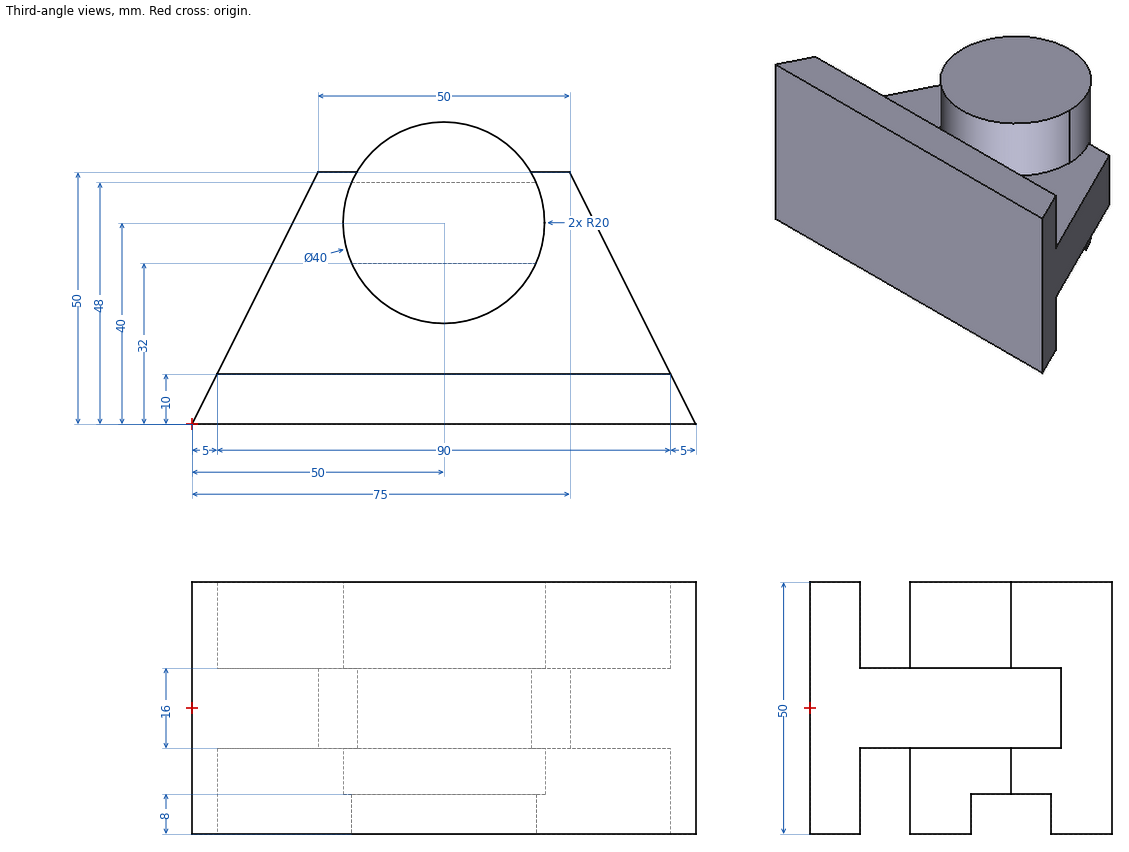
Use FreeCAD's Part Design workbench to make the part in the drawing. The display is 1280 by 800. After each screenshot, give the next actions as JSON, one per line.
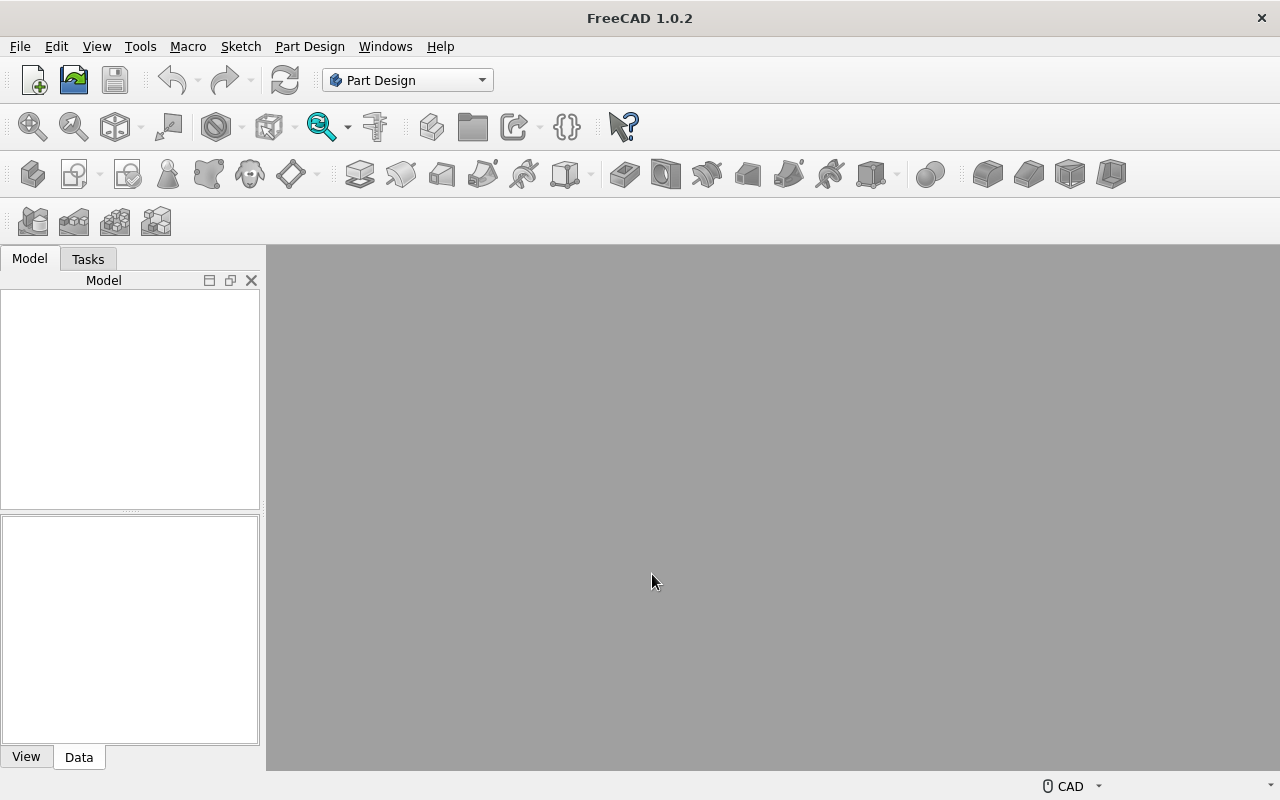
{"action": "left_click", "coordinate": [33, 80]}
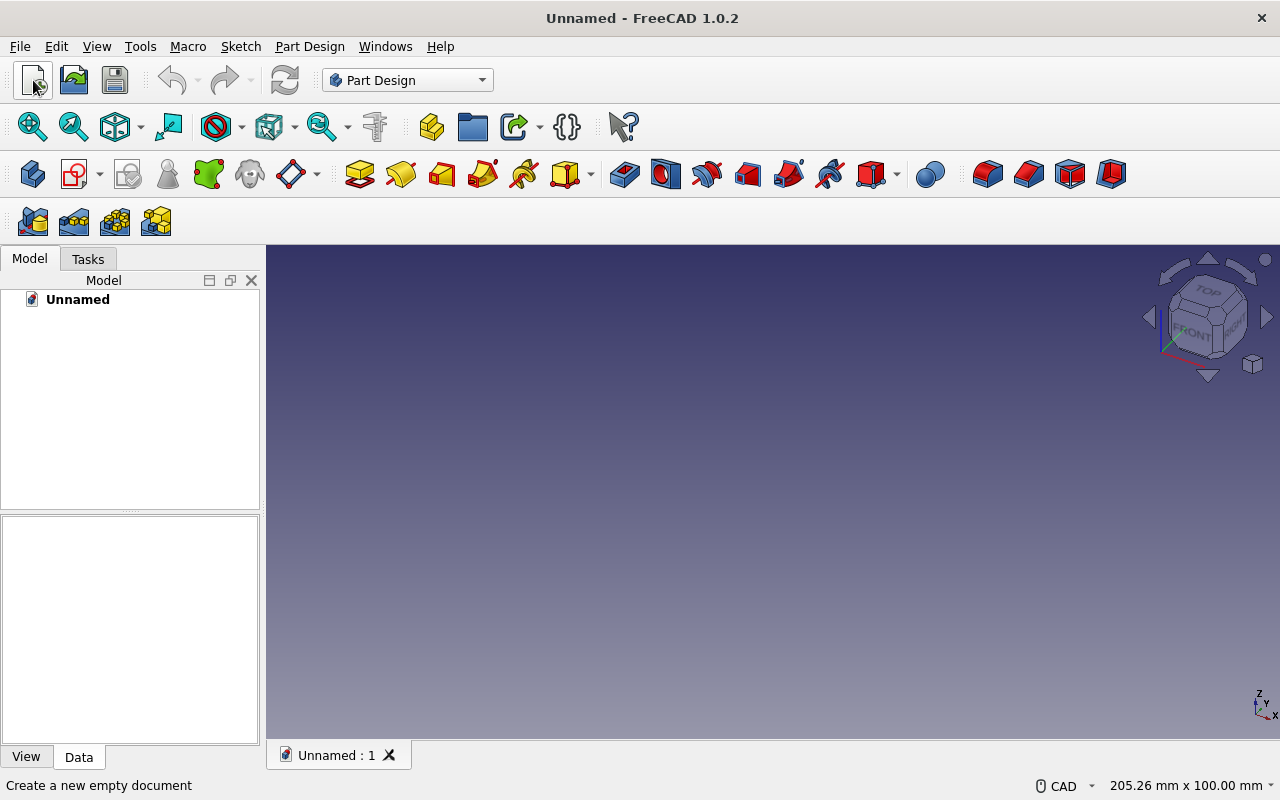
{"action": "left_click", "coordinate": [74, 174]}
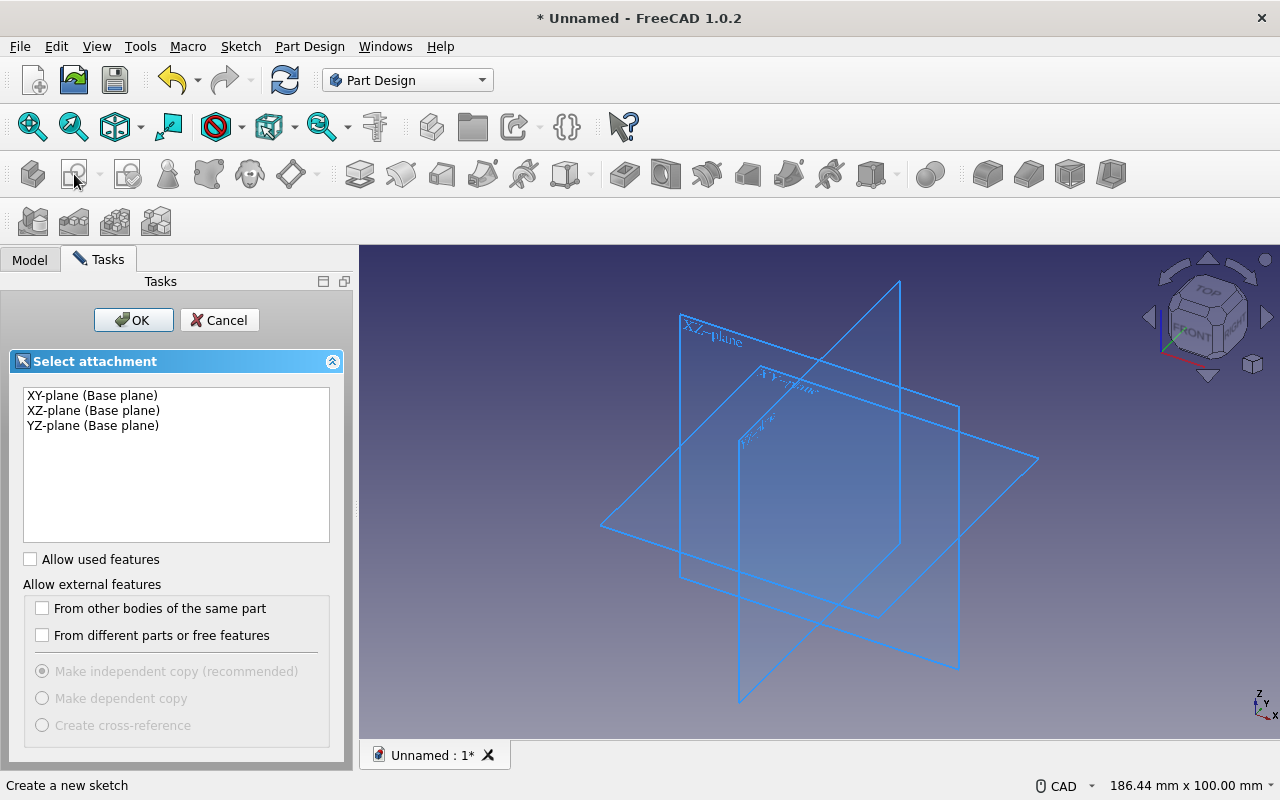
{"action": "left_click", "coordinate": [84, 396]}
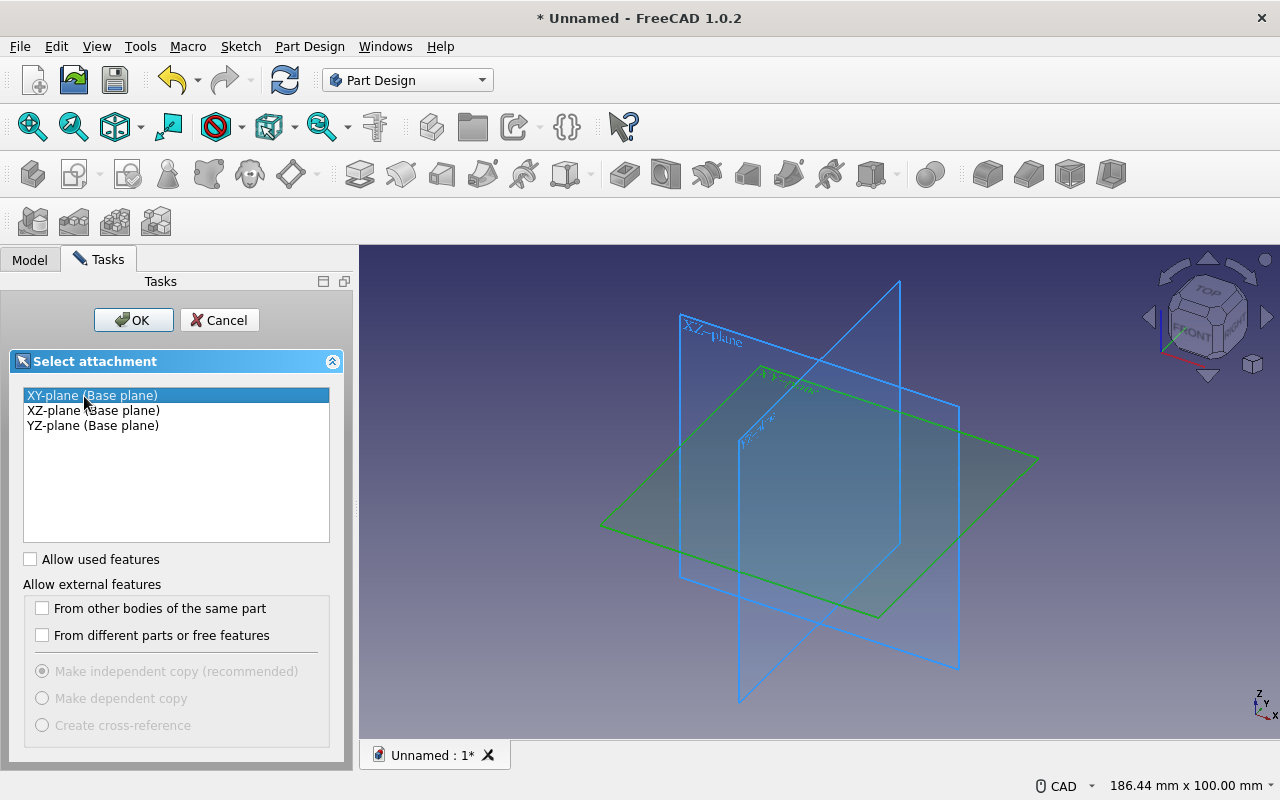
{"action": "left_click", "coordinate": [134, 320]}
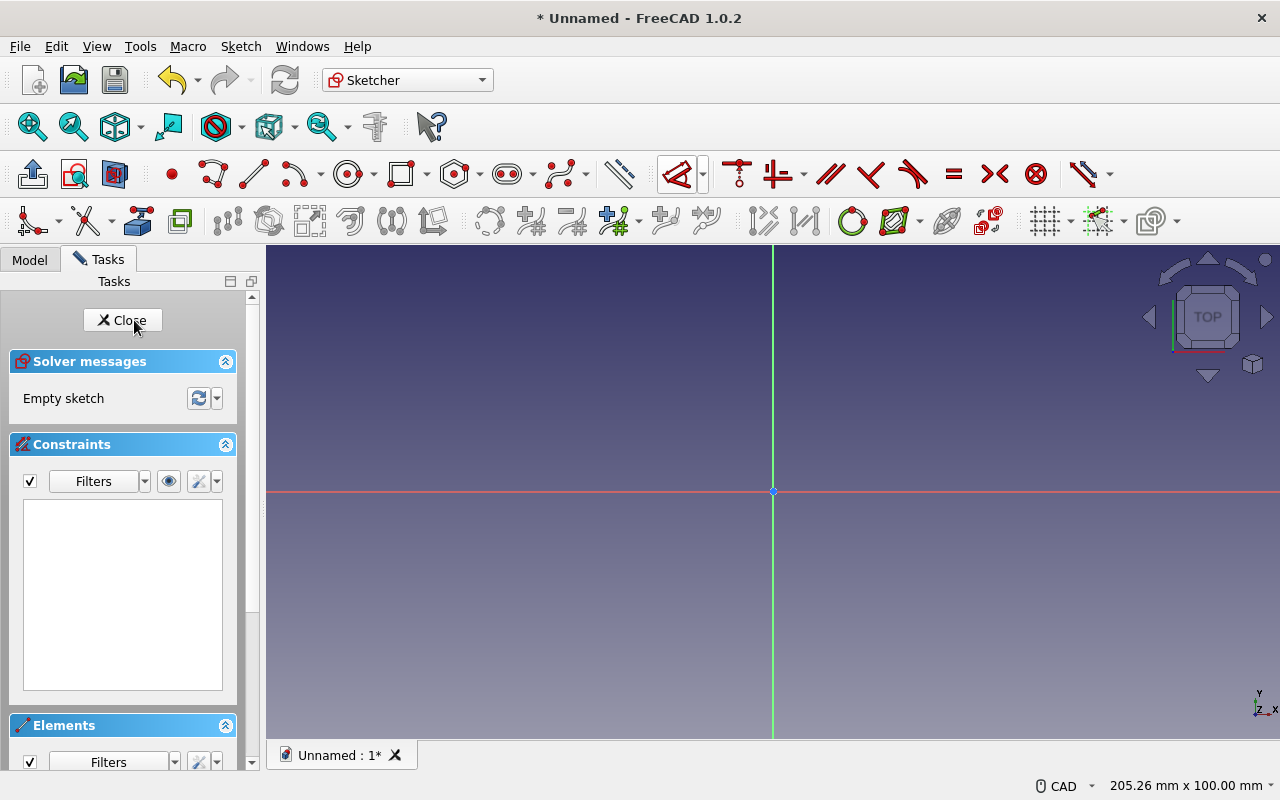
{"action": "scroll", "coordinate": [294, 542], "scroll_direction": "down", "scroll_amount": 2}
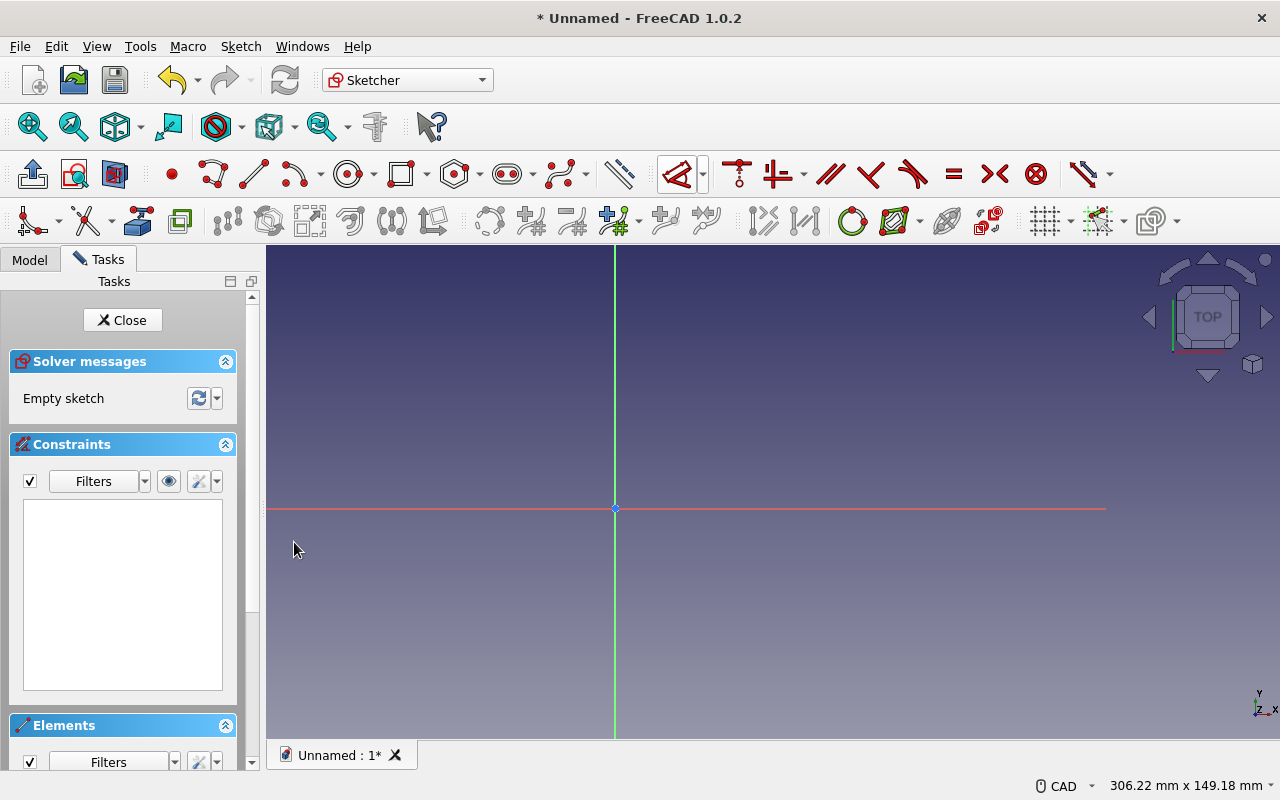
{"action": "scroll", "coordinate": [873, 492], "scroll_direction": "up", "scroll_amount": 3}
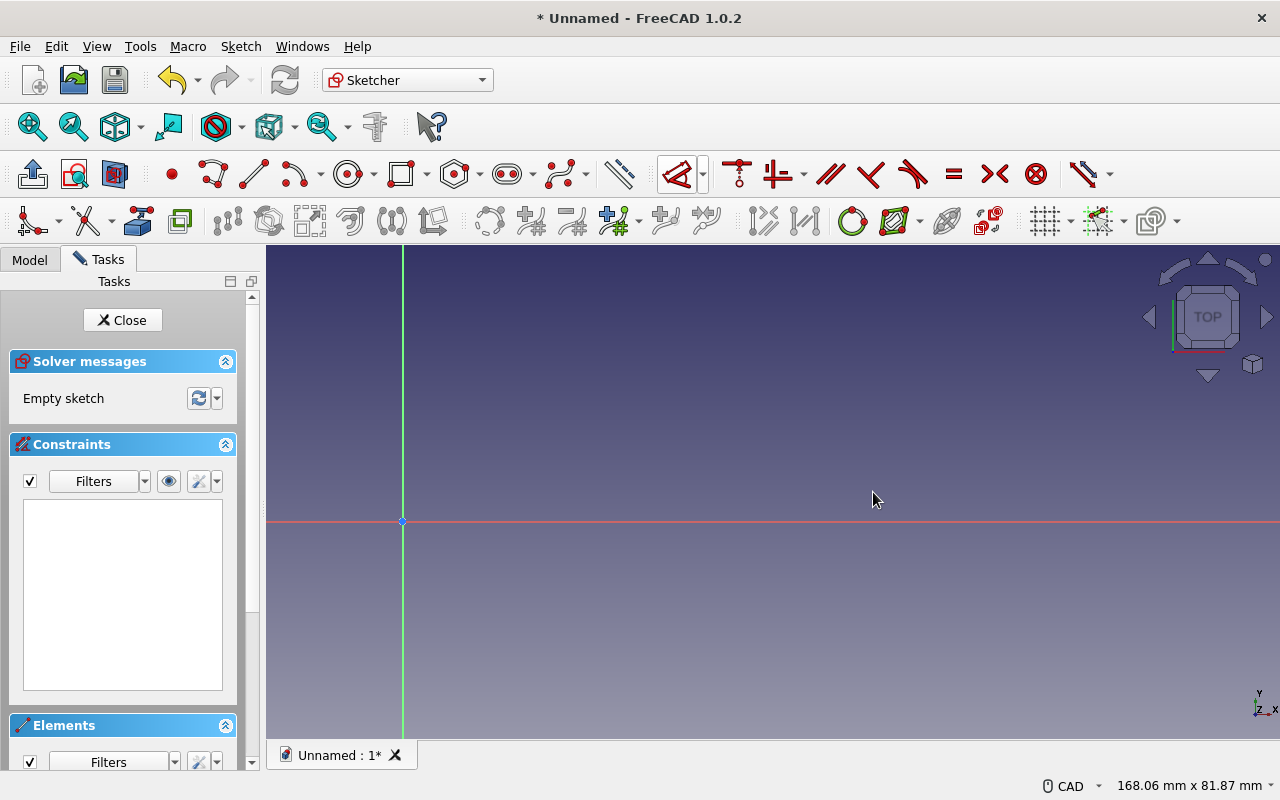
{"action": "left_click", "coordinate": [213, 174]}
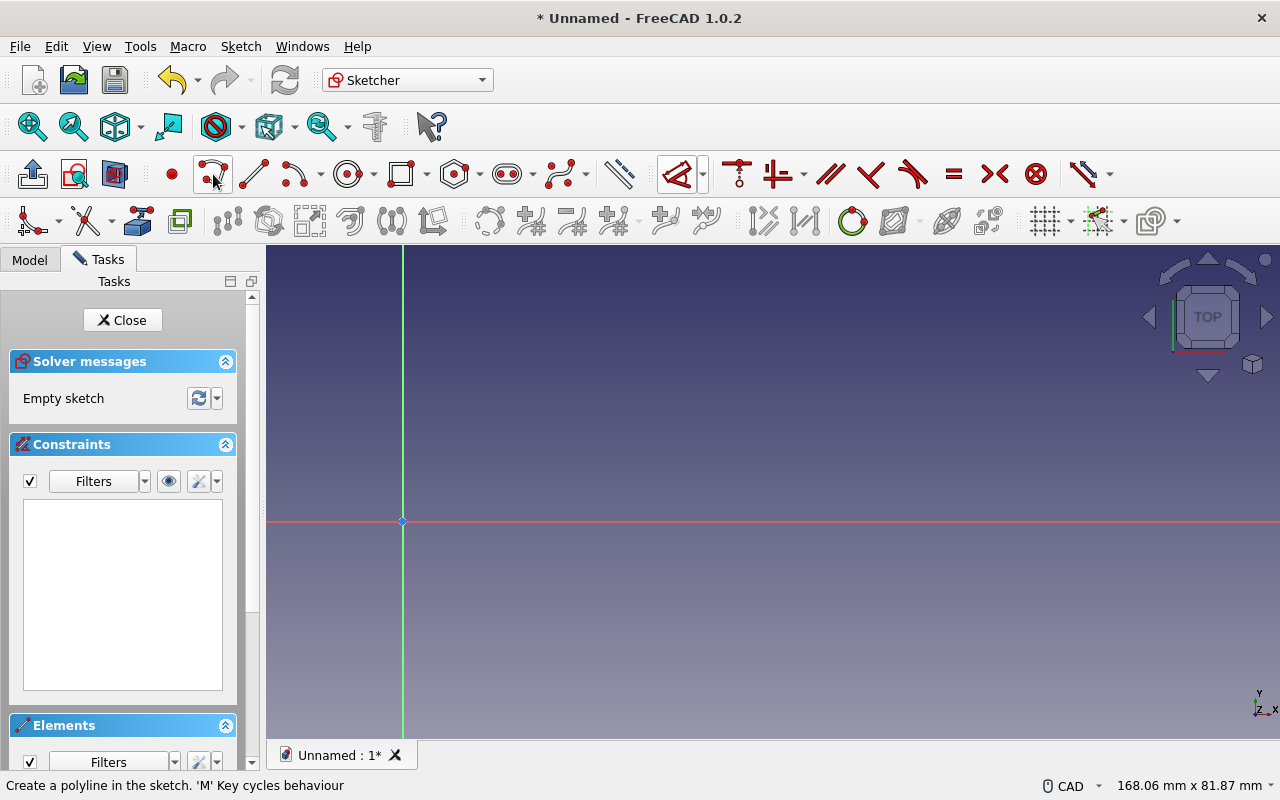
{"action": "left_click", "coordinate": [403, 522]}
{"action": "left_click", "coordinate": [1006, 513]}
{"action": "left_click", "coordinate": [976, 462]}
{"action": "left_click", "coordinate": [433, 462]}
{"action": "left_click", "coordinate": [403, 522]}
{"action": "key", "text": "Escape"}
{"action": "key", "text": "Escape"}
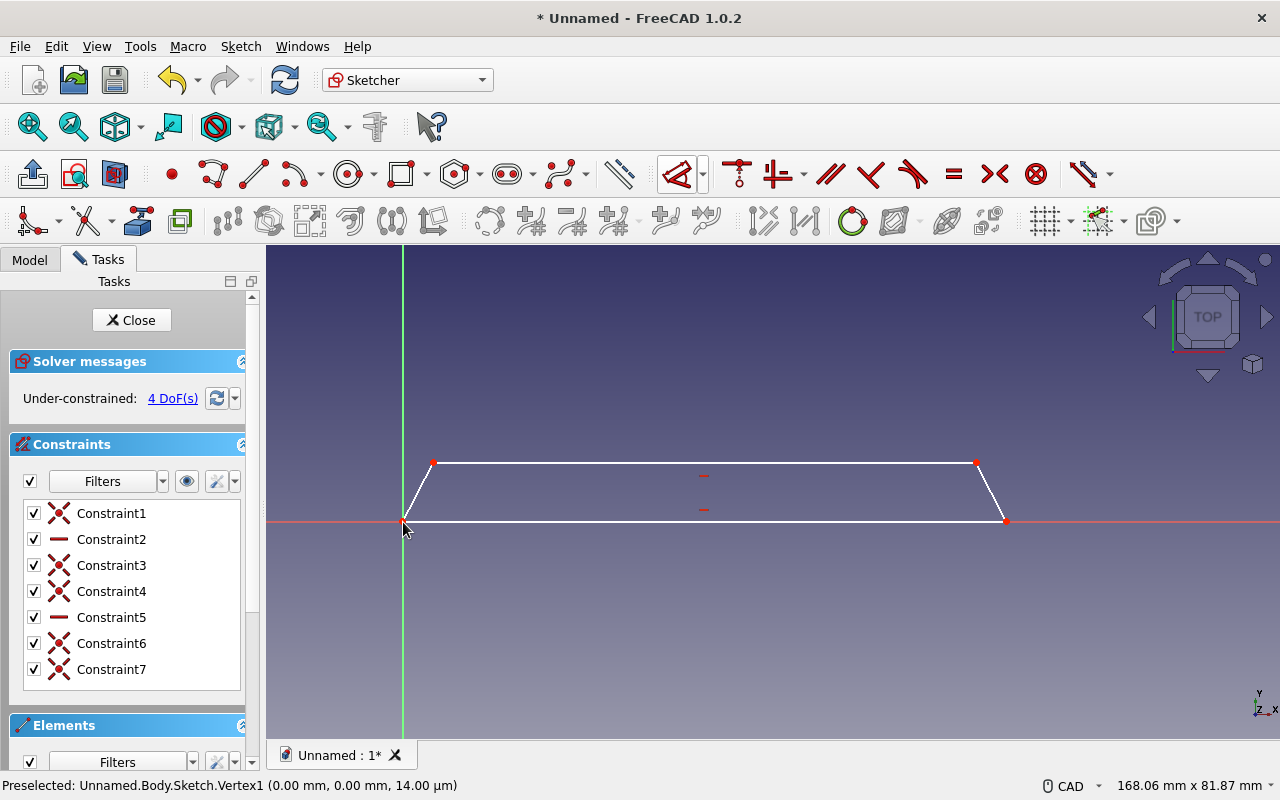
{"action": "left_click", "coordinate": [676, 174]}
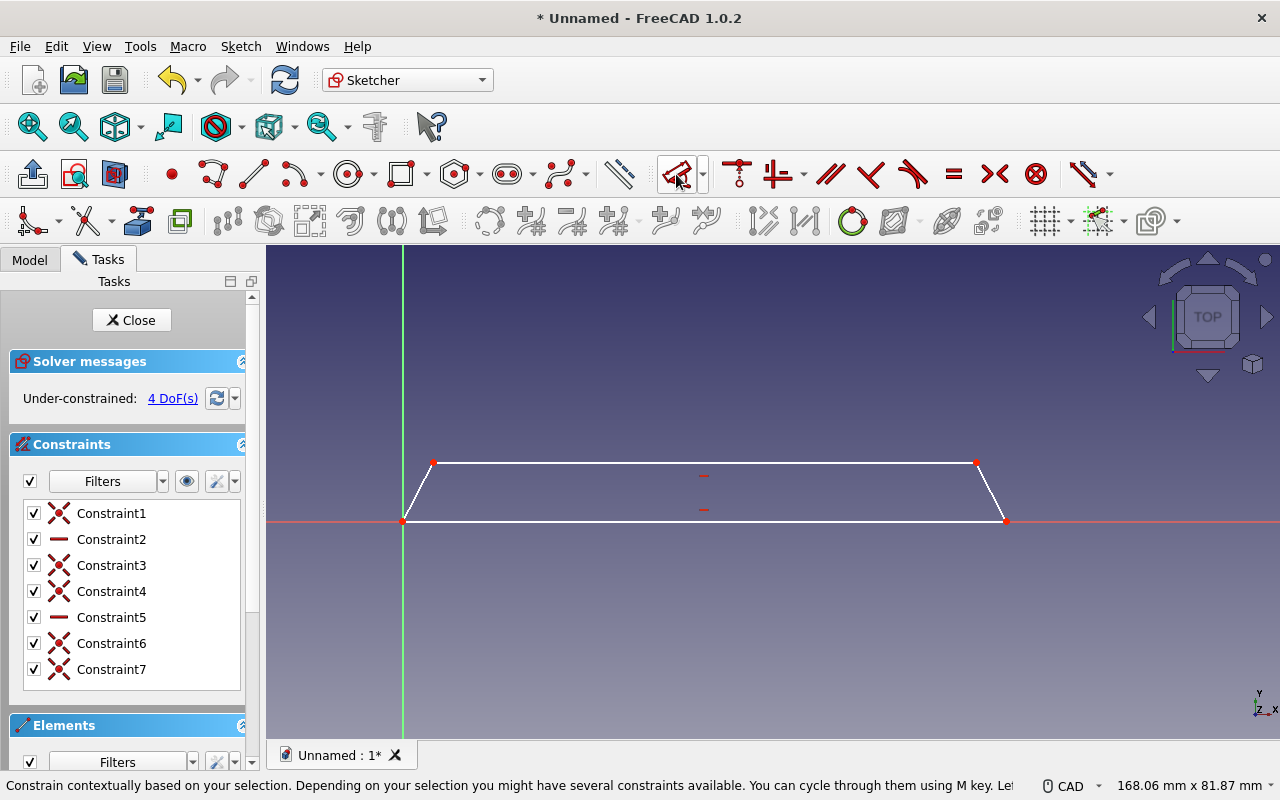
{"action": "left_click", "coordinate": [813, 463]}
{"action": "left_click", "coordinate": [704, 429]}